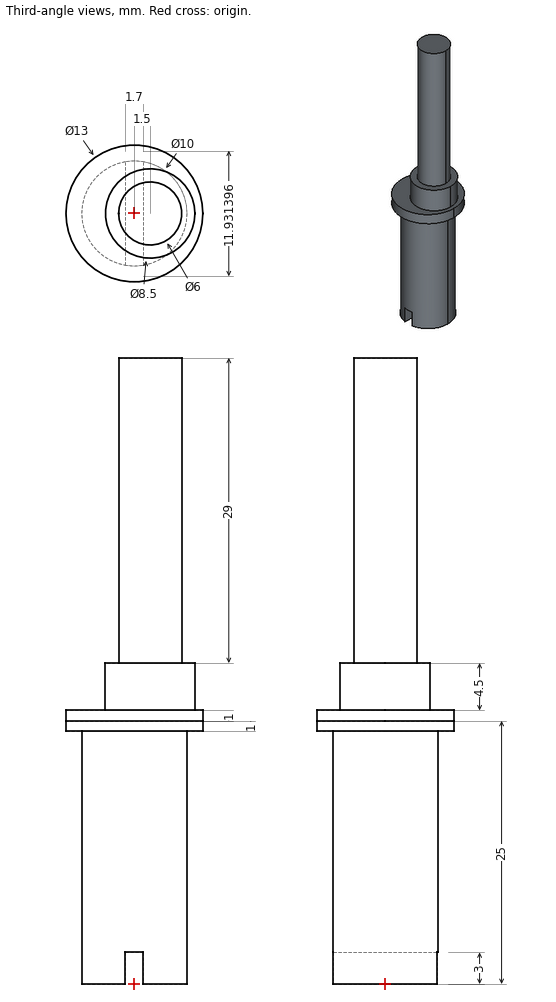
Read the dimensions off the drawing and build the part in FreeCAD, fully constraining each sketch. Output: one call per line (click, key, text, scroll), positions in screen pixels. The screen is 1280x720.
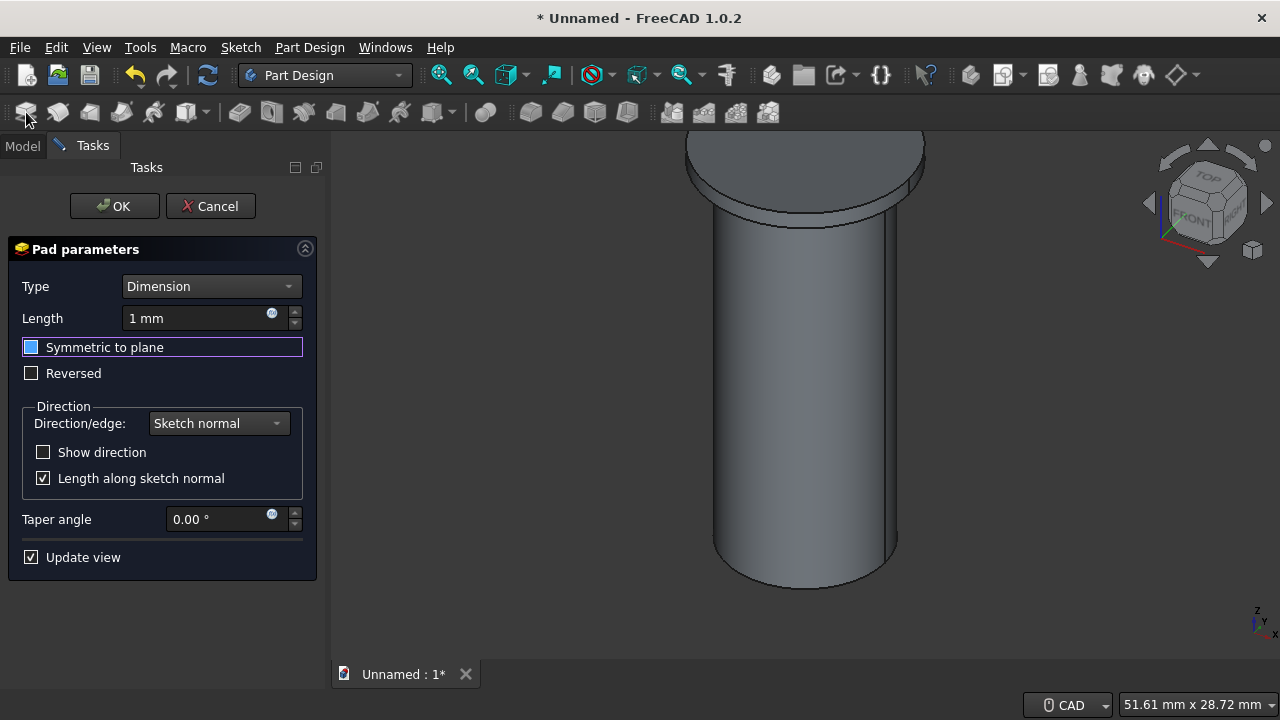
click(115, 206)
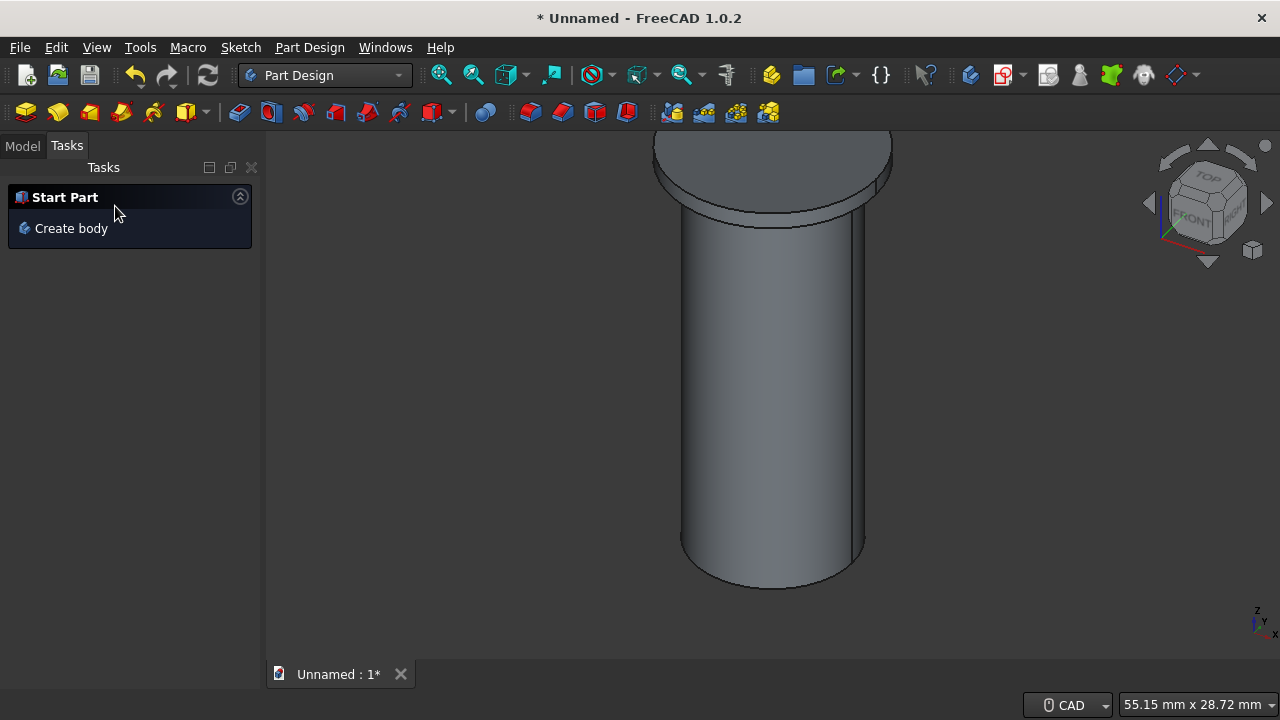
click(442, 76)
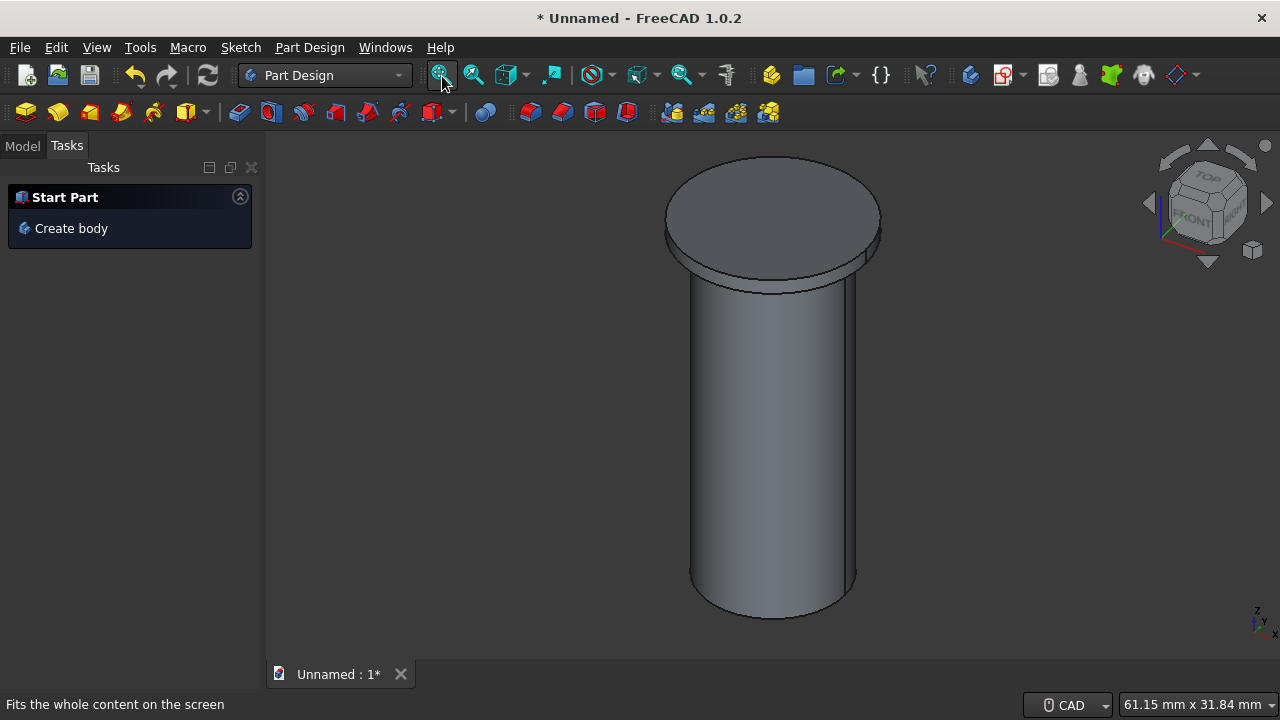
click(773, 217)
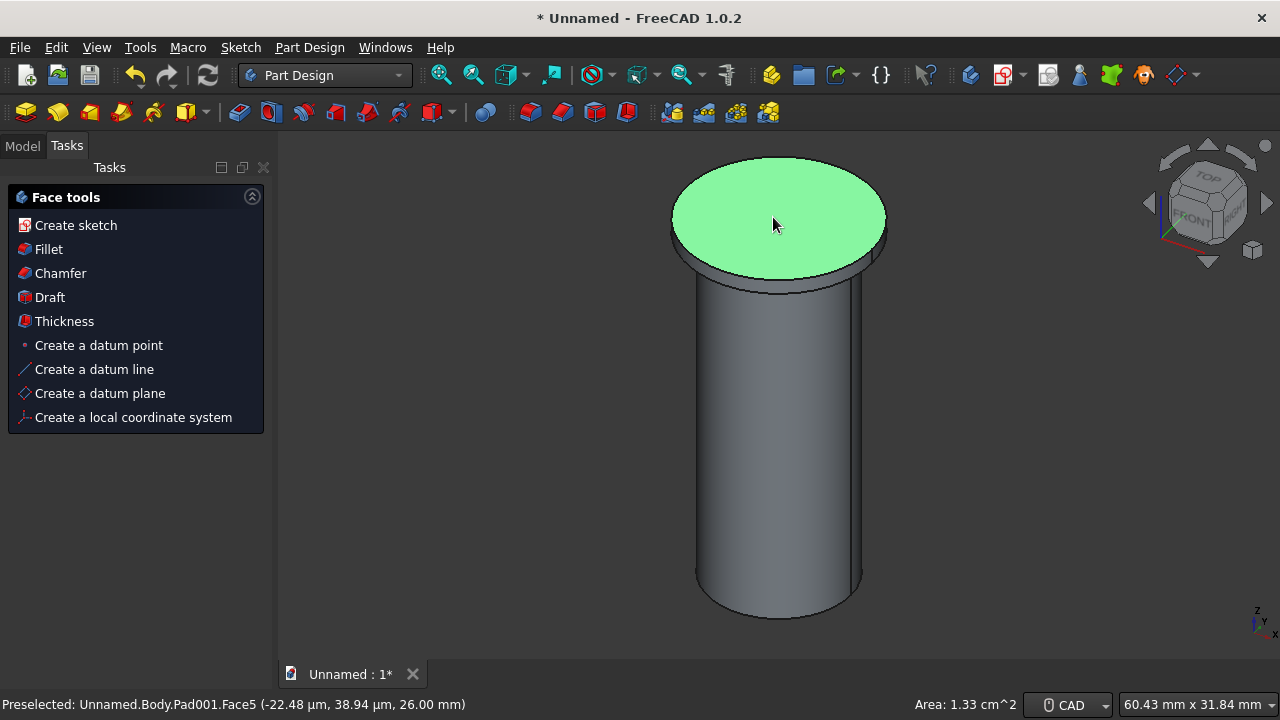
click(1004, 76)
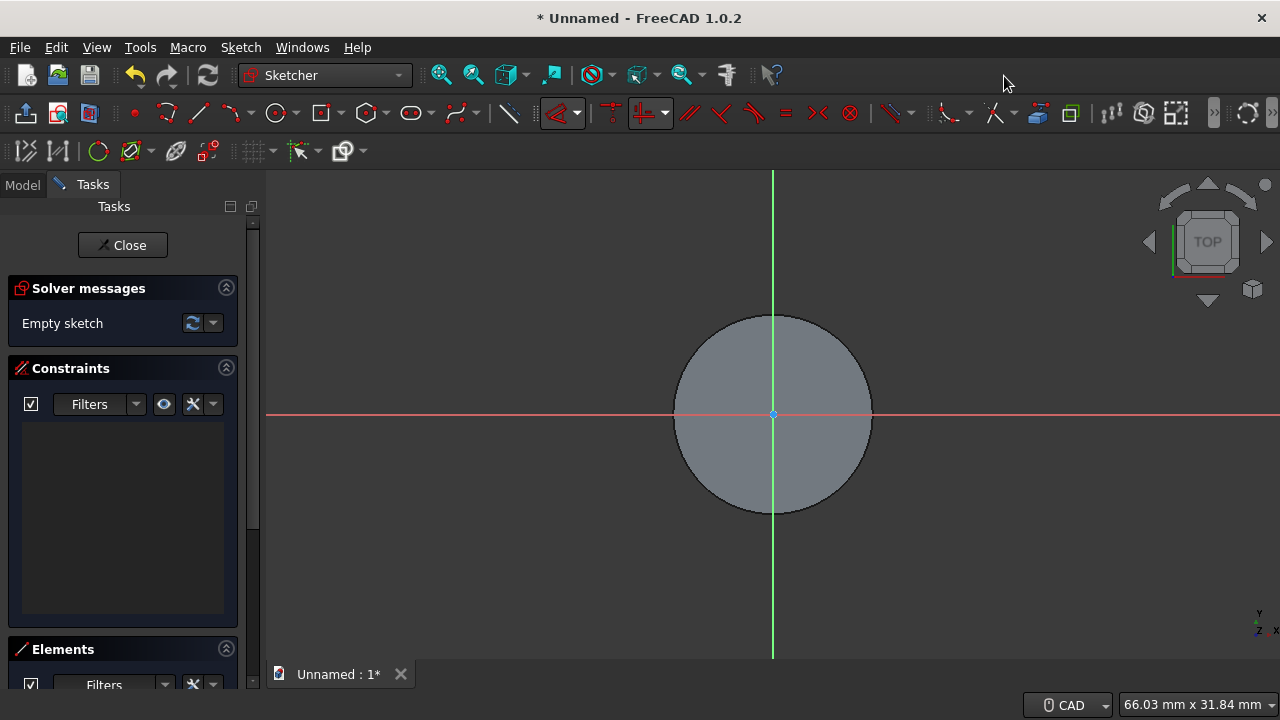
scroll(871, 414, up, 4)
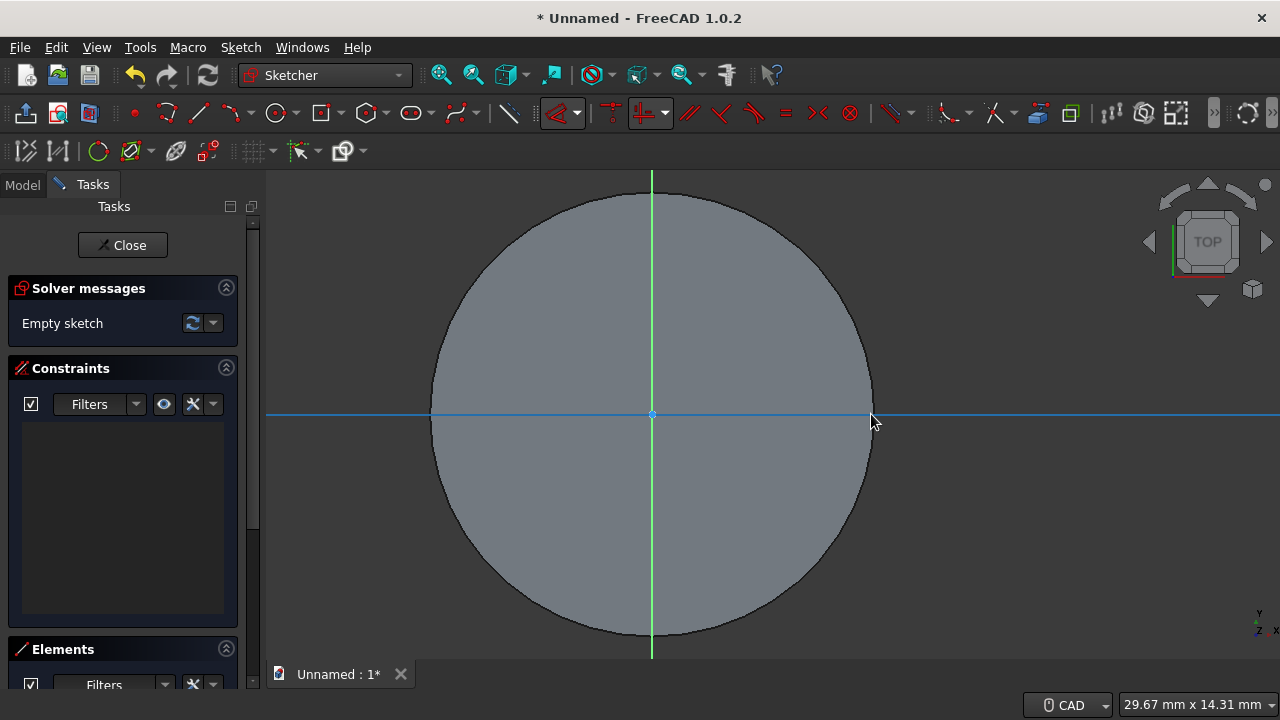
click(276, 114)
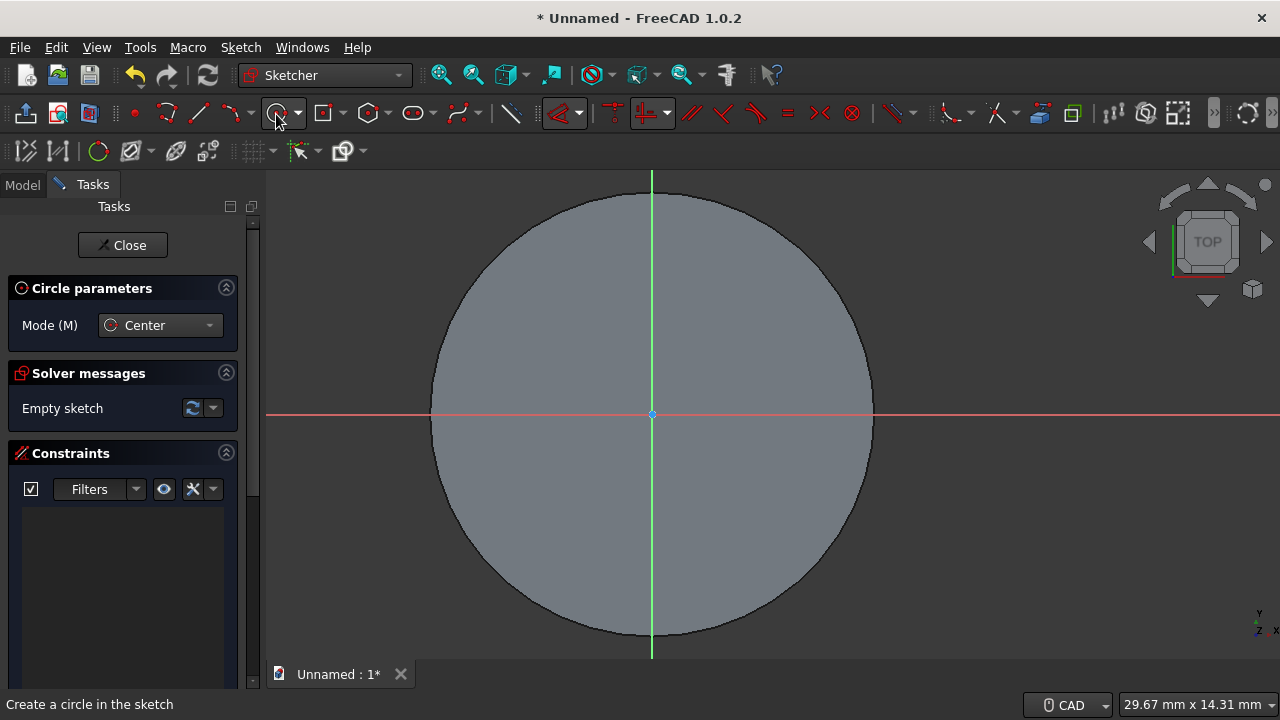
click(703, 414)
move(806, 312)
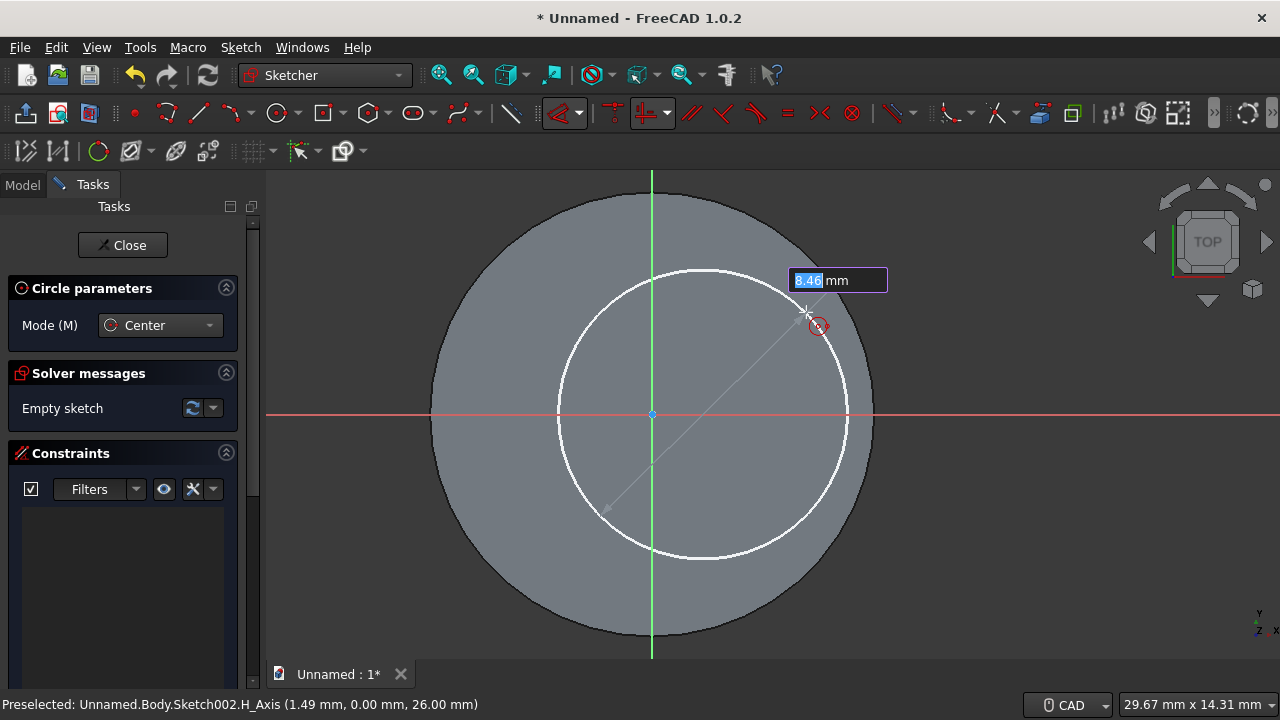
text(8.5)
key(Return)
key(Escape)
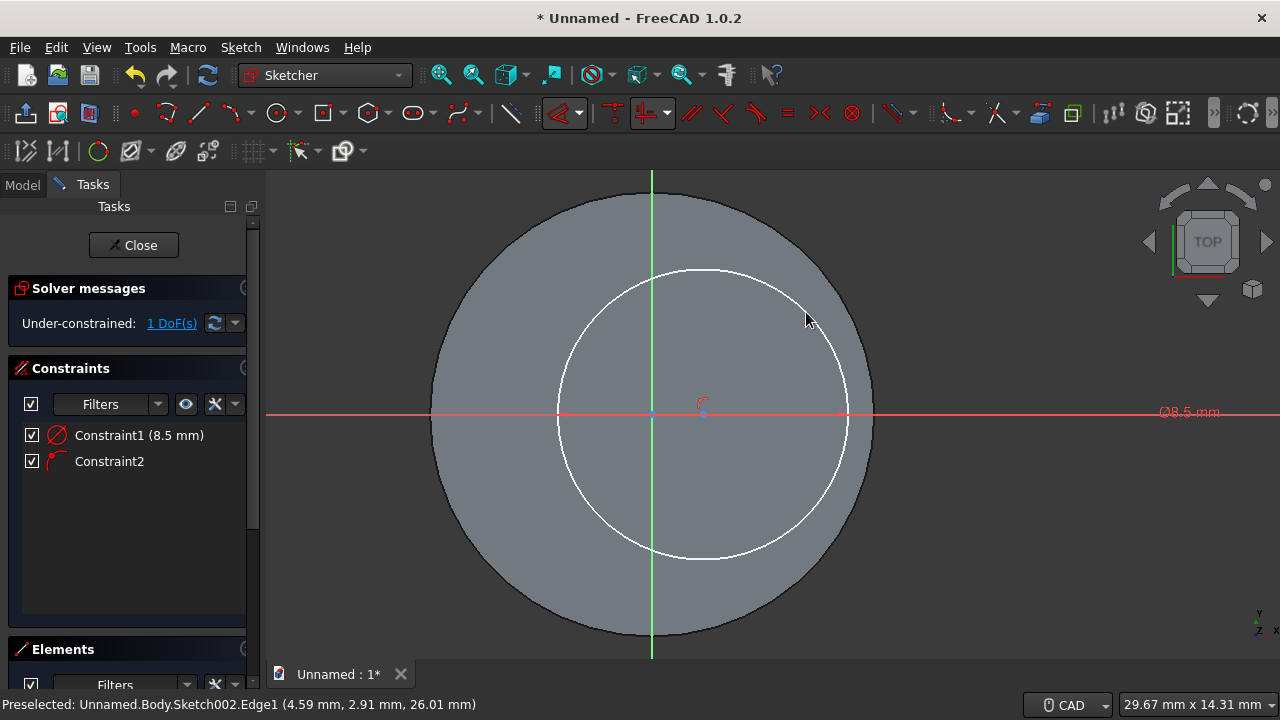
click(703, 414)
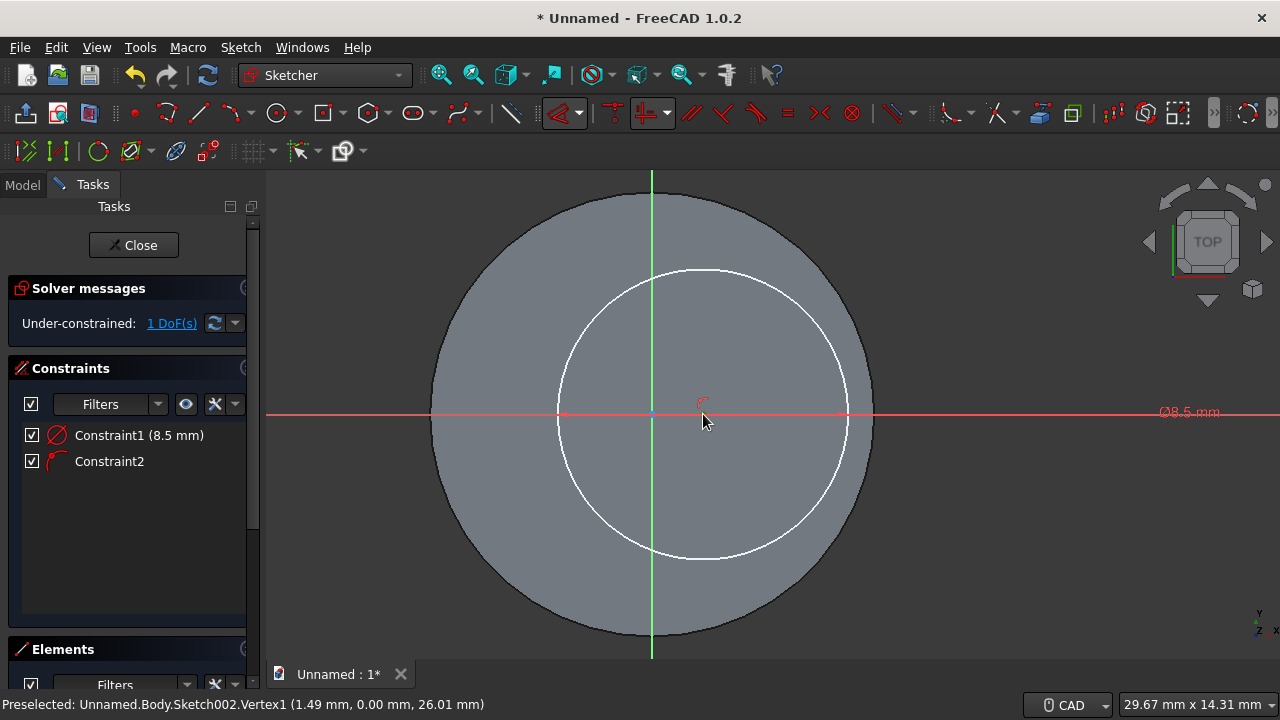
click(582, 114)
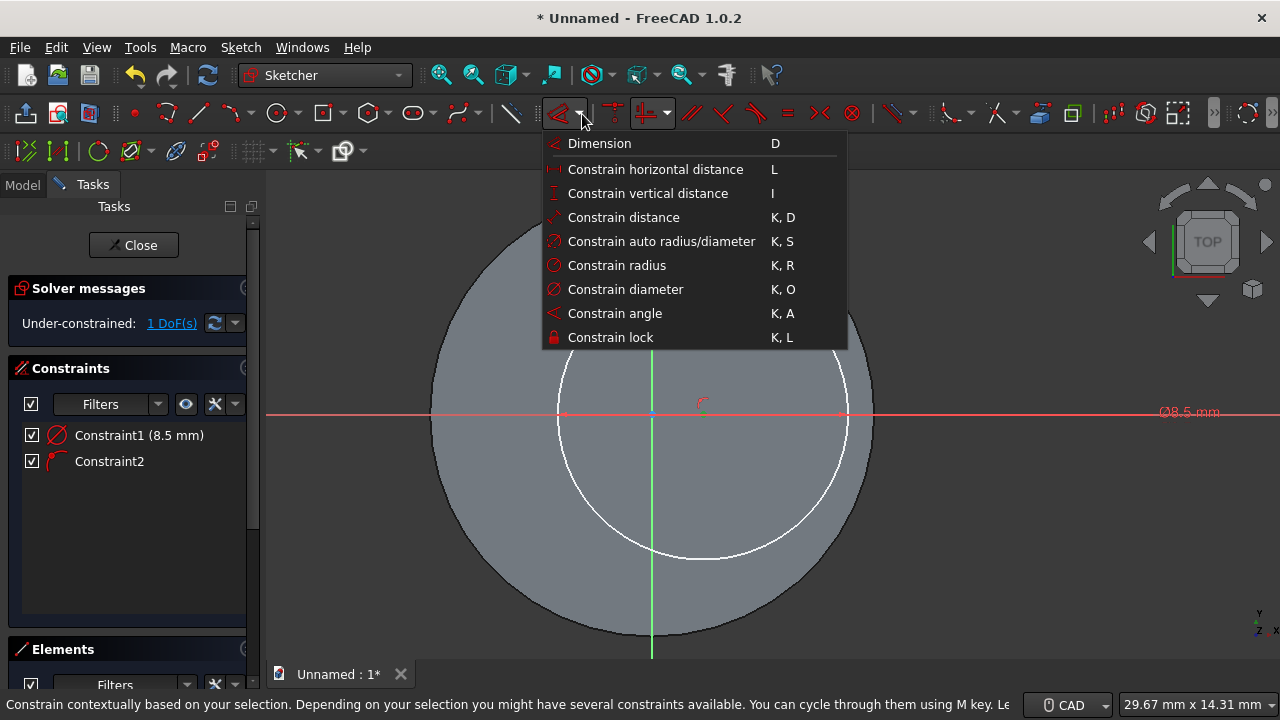
click(695, 169)